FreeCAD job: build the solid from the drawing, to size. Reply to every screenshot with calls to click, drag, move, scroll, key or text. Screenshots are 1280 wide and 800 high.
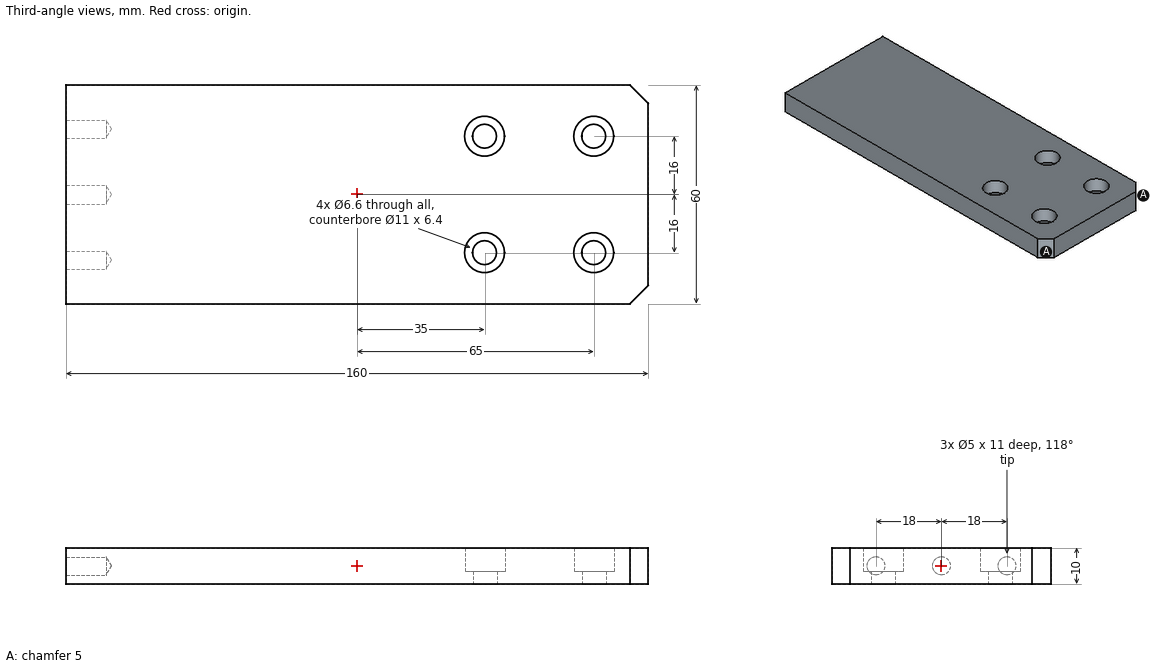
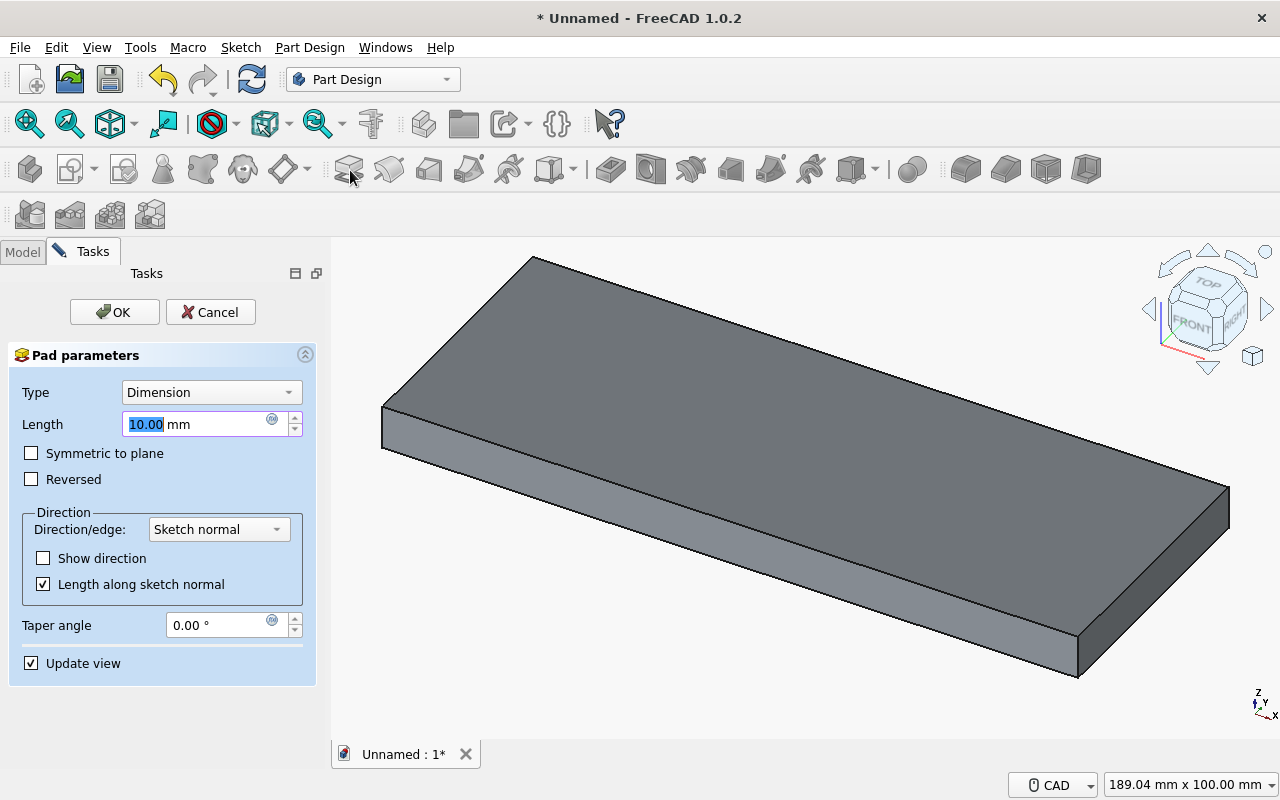
text(10)
key(Tab)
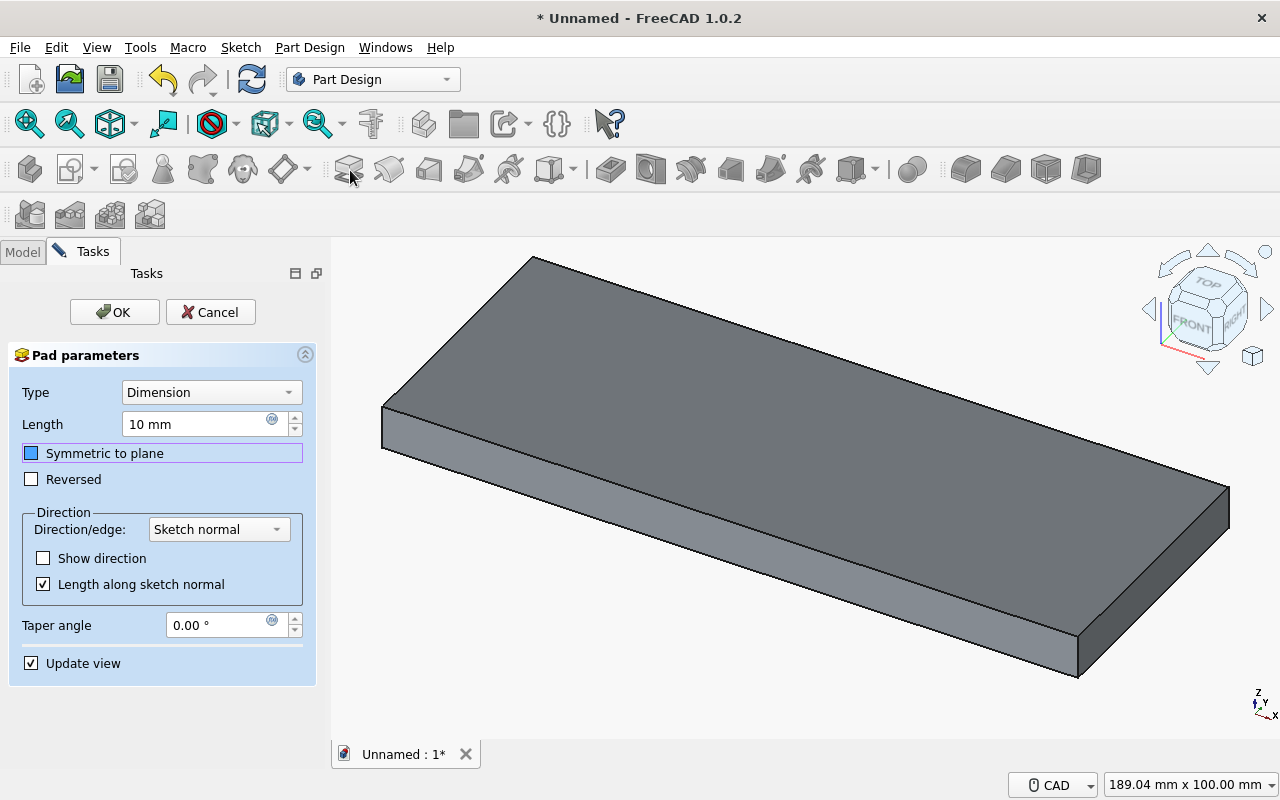
click(30, 453)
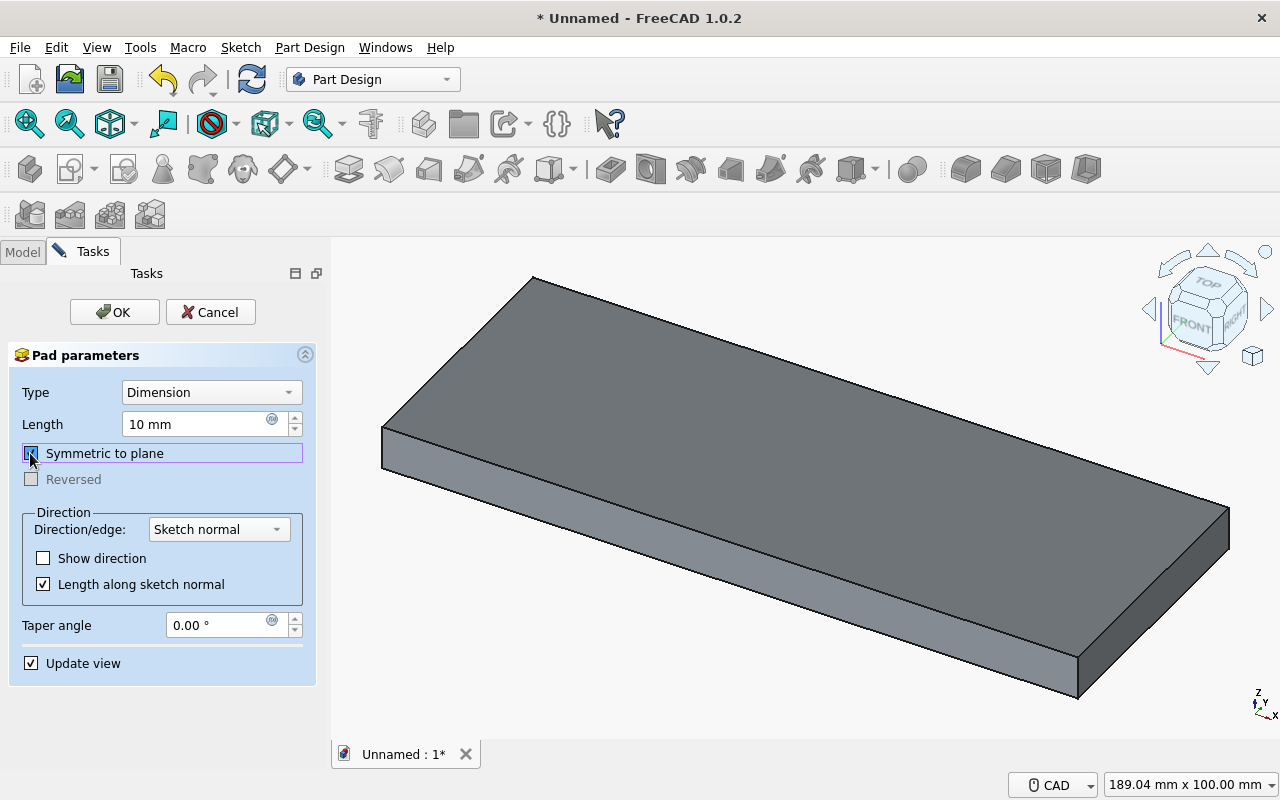
click(115, 312)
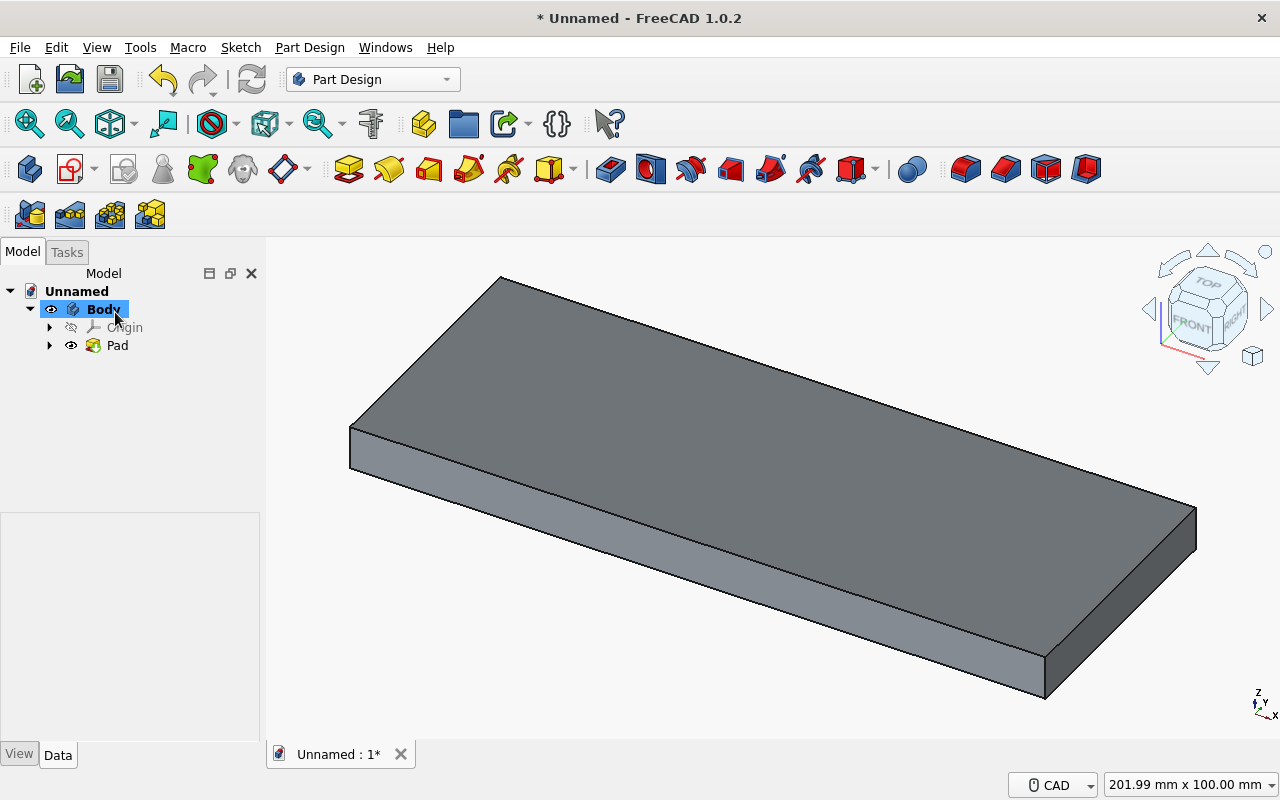
click(972, 532)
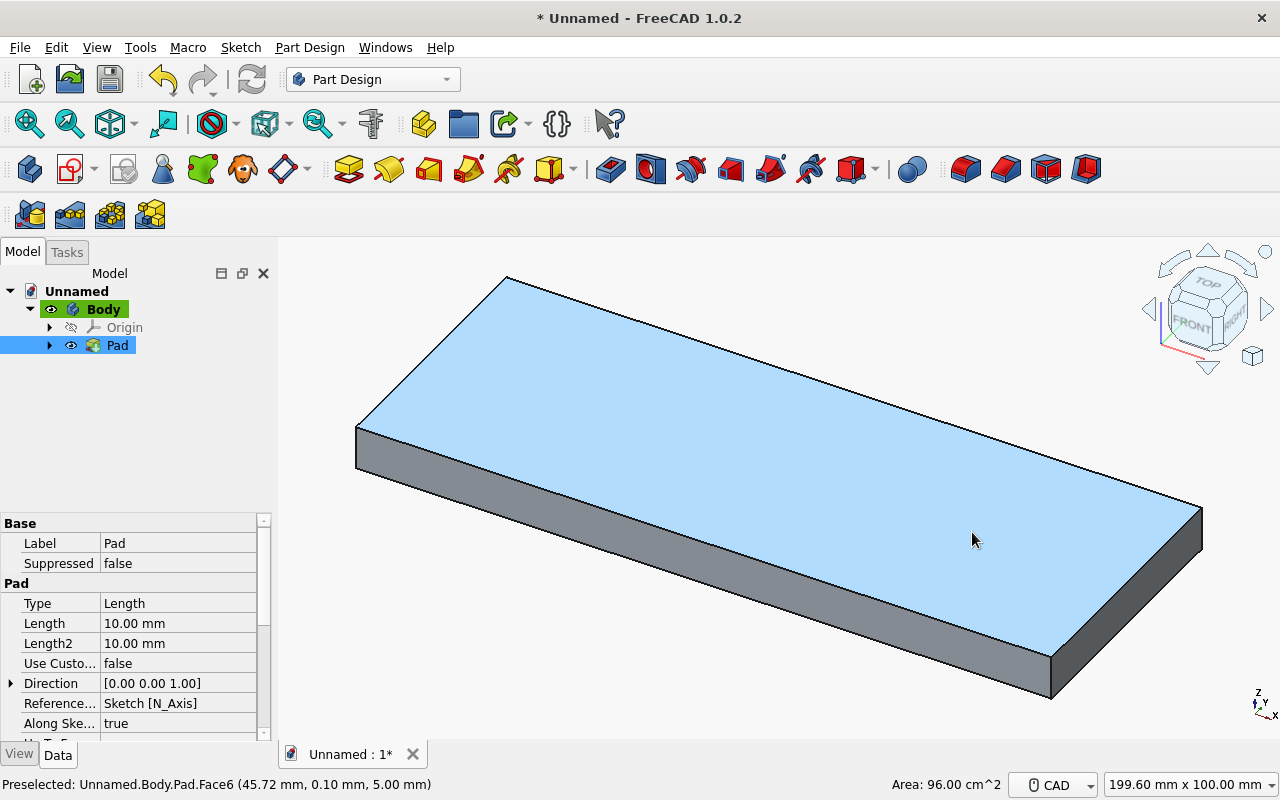
click(70, 170)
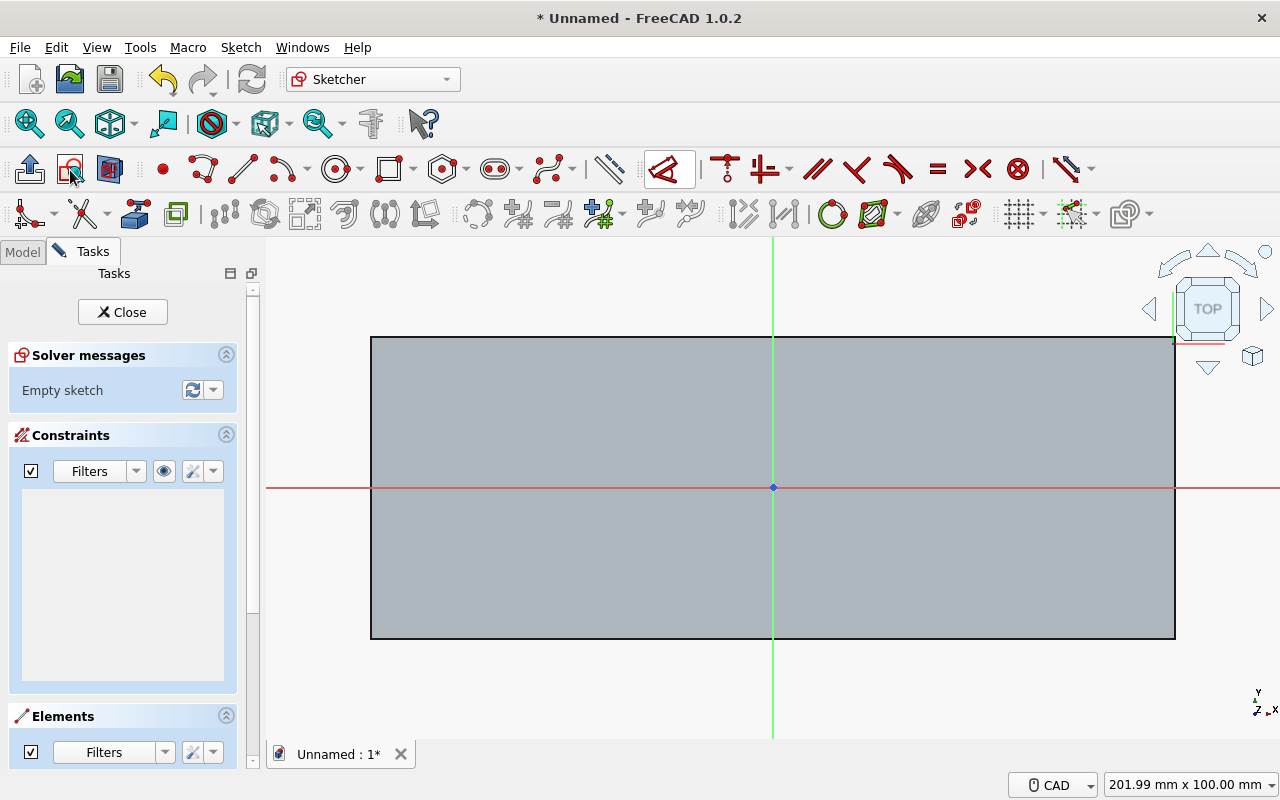
scroll(294, 488, down, 1)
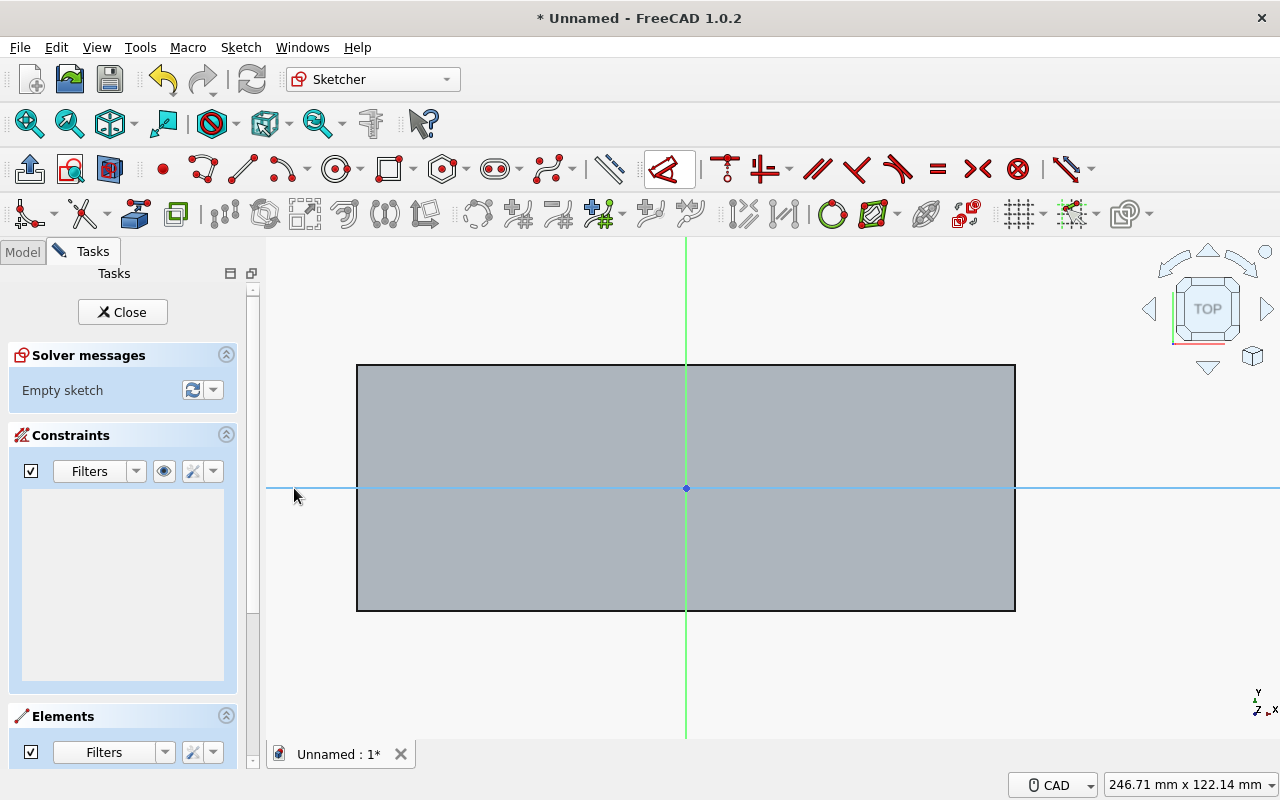
scroll(975, 488, up, 3)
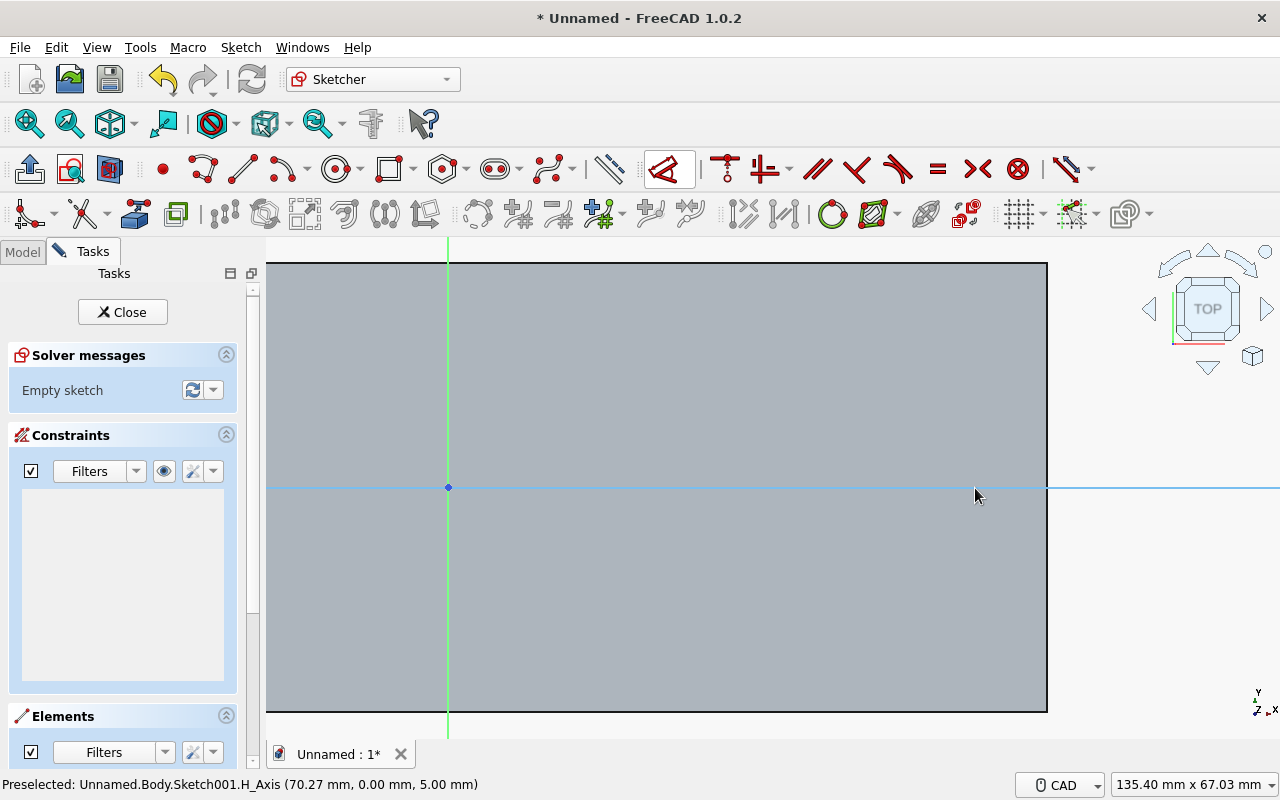
key(g)
key(c)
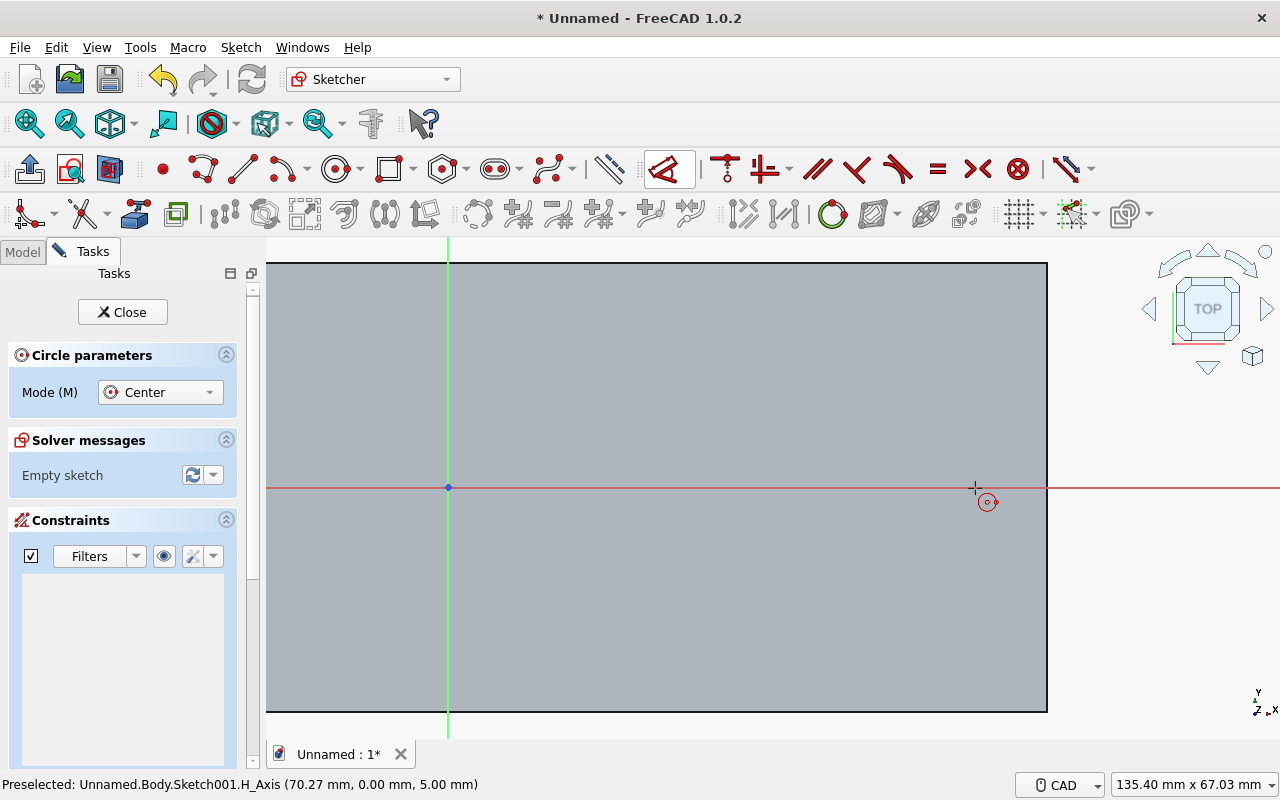
click(710, 608)
move(728, 590)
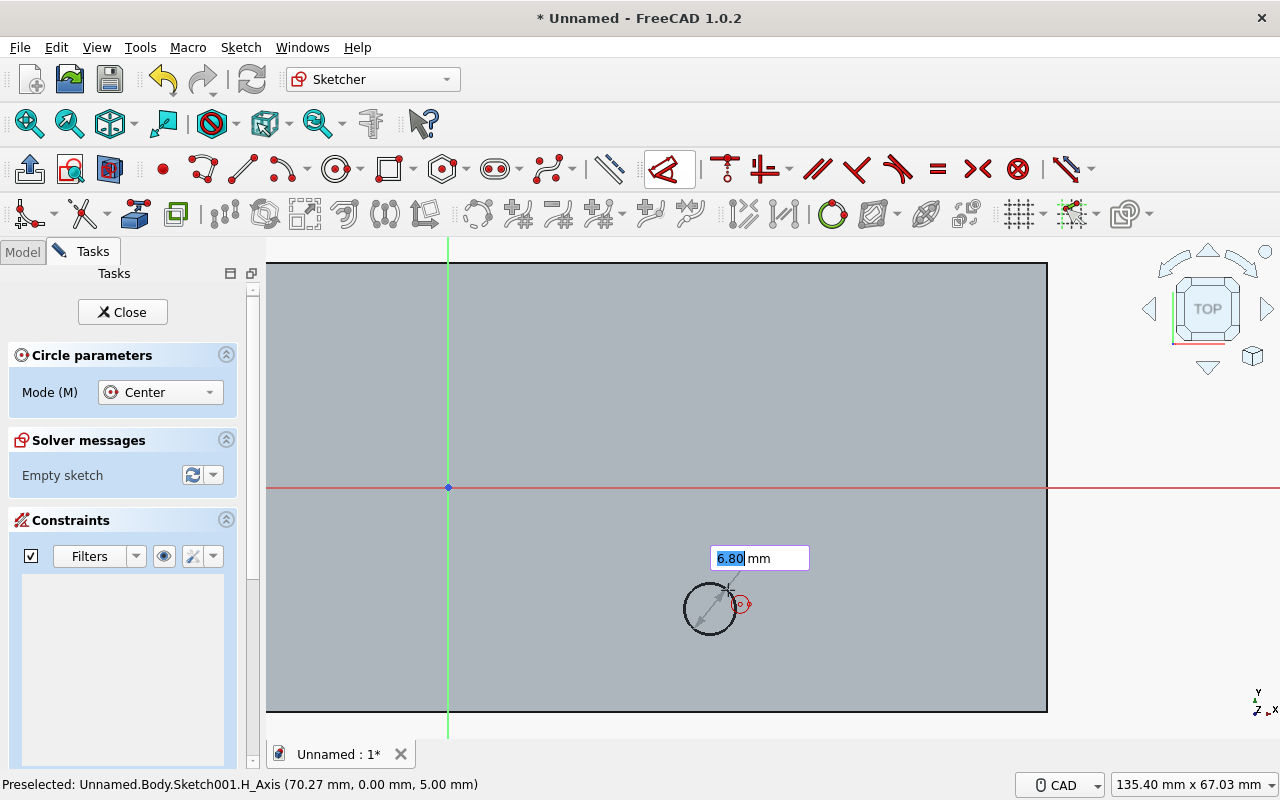
text(6.6)
key(Return)